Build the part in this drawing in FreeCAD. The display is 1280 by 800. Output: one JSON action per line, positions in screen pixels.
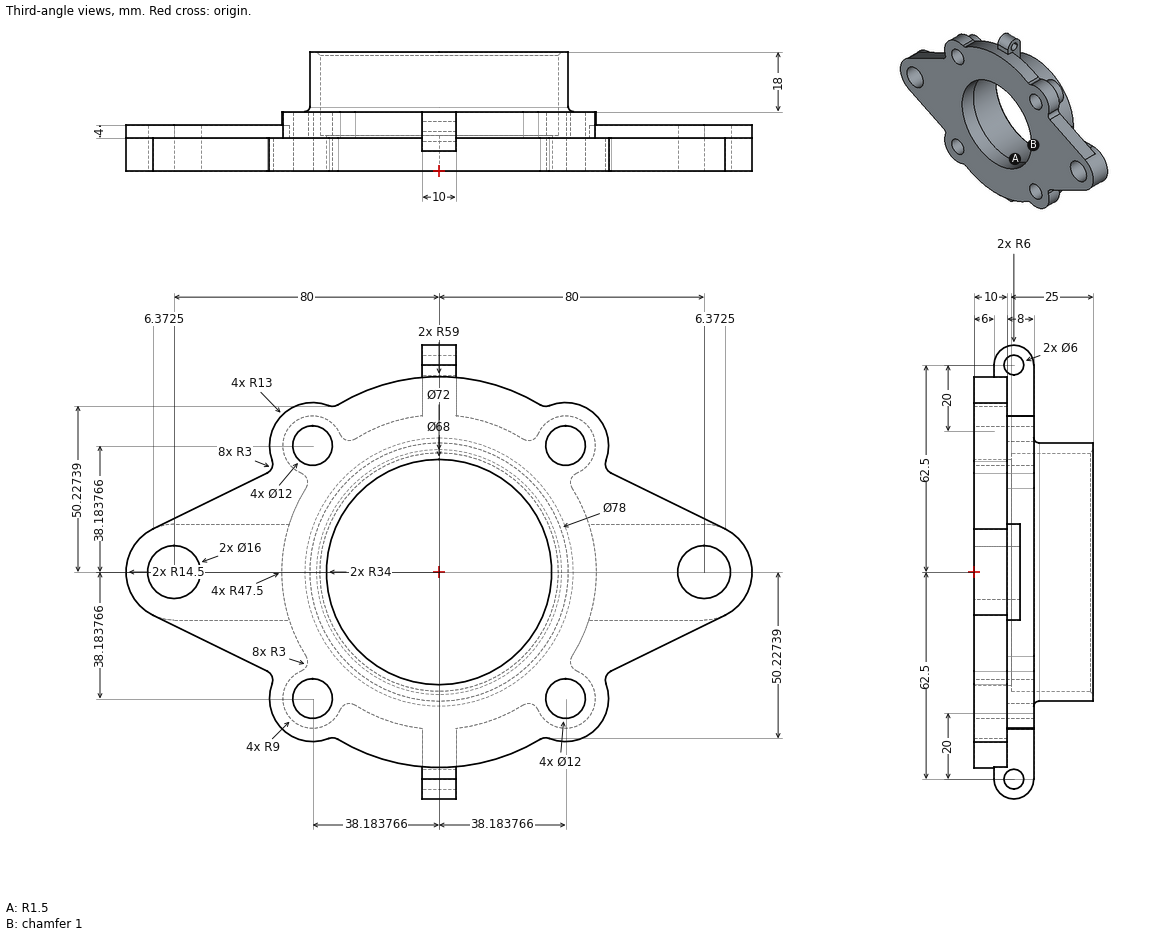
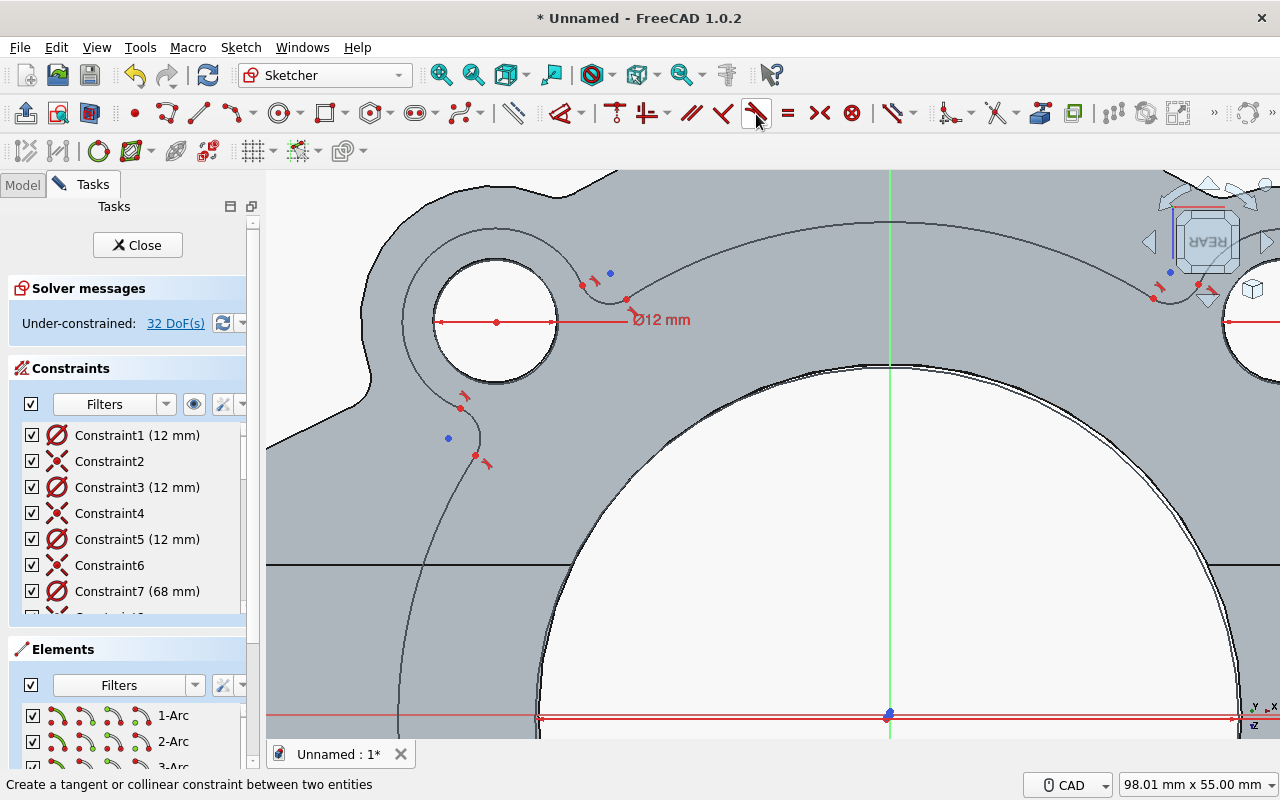
{"action": "left_click", "coordinate": [638, 471]}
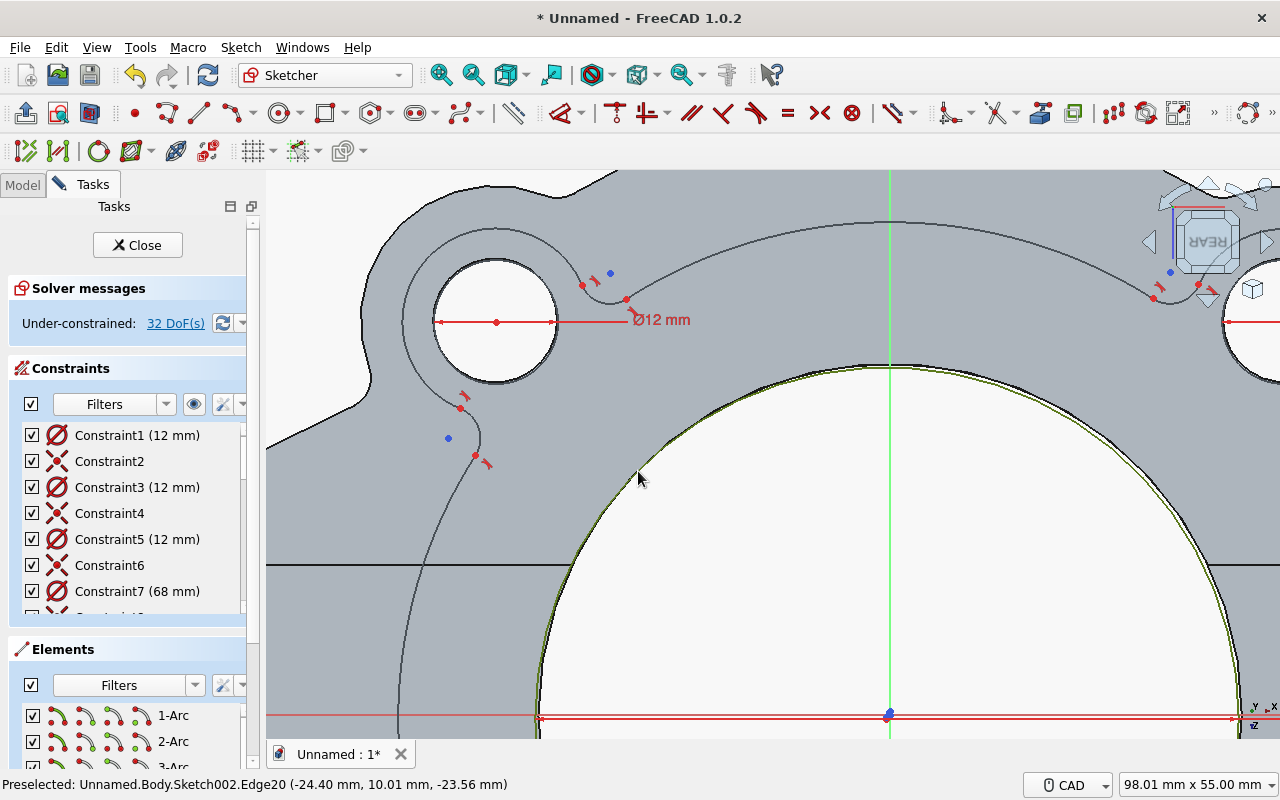
{"action": "scroll", "coordinate": [596, 303], "scroll_direction": "down", "scroll_amount": 5}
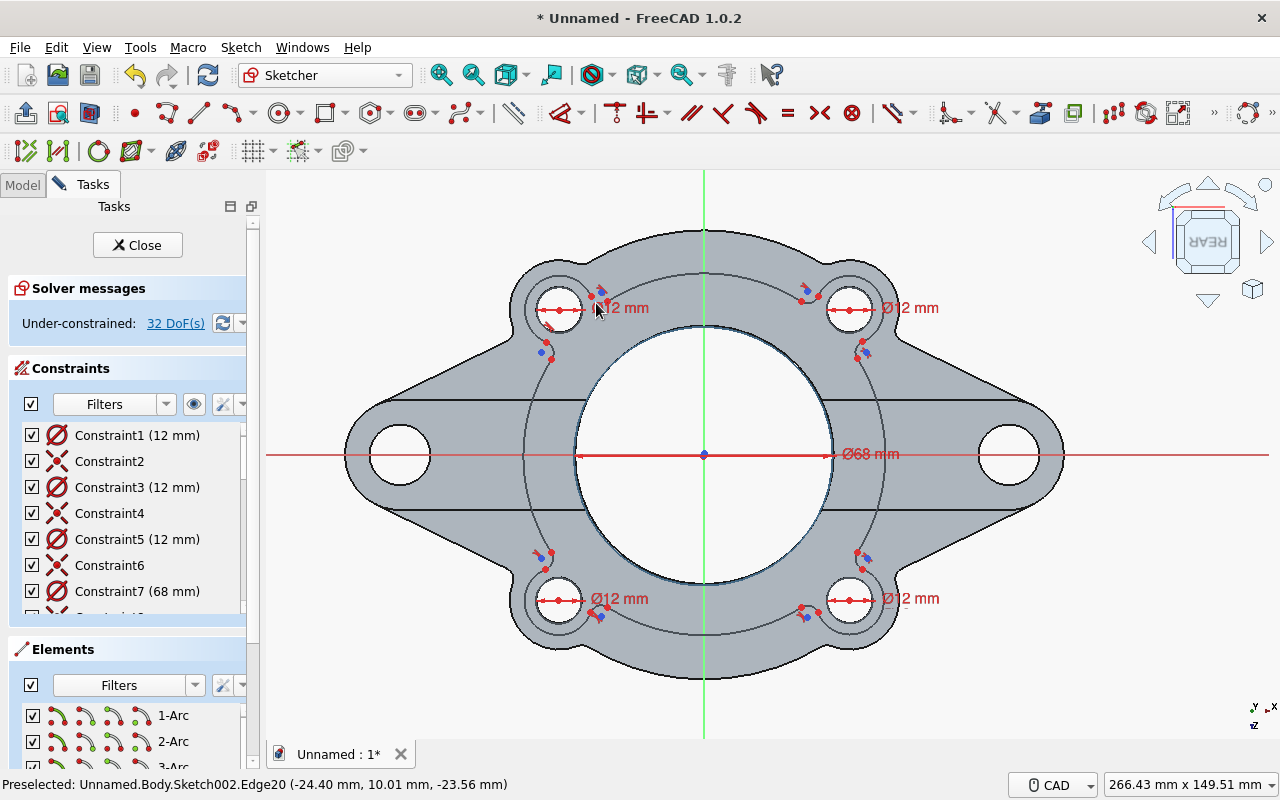
{"action": "left_click", "coordinate": [664, 631]}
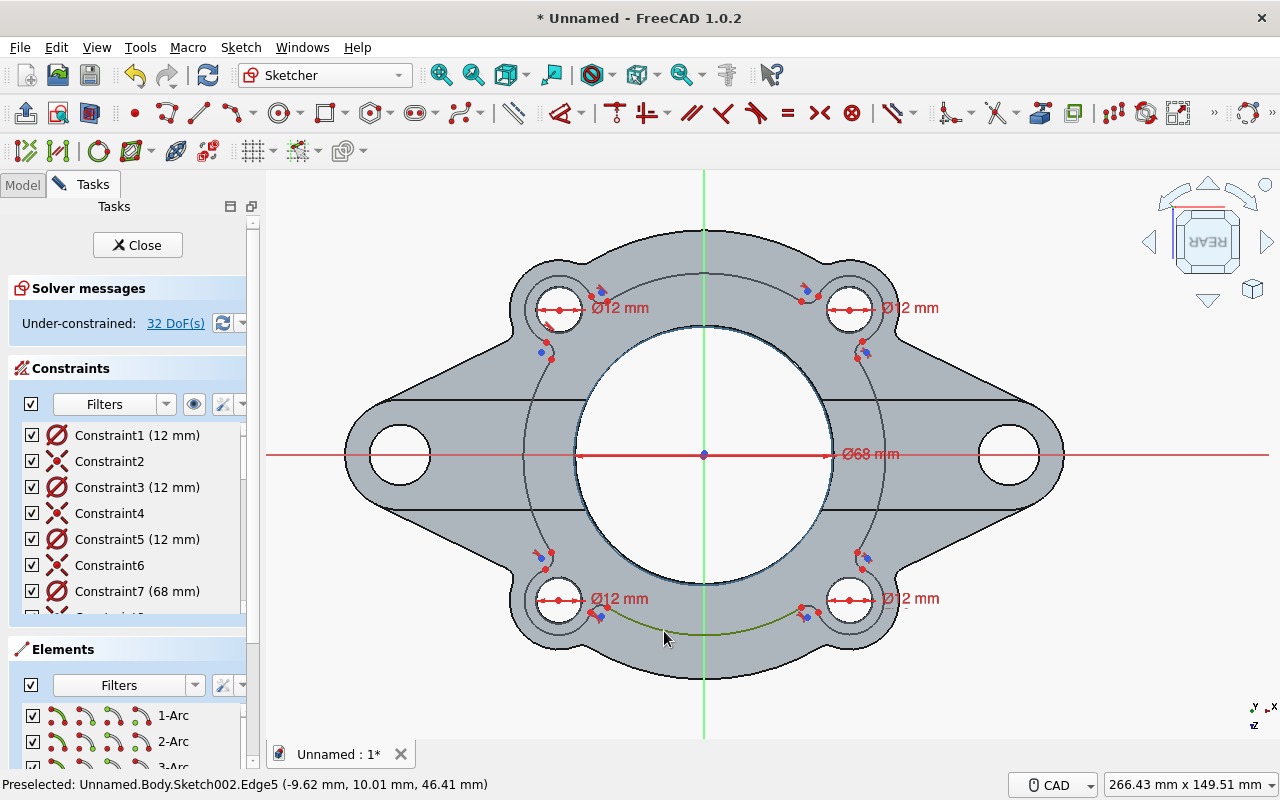
{"action": "left_click", "coordinate": [616, 114]}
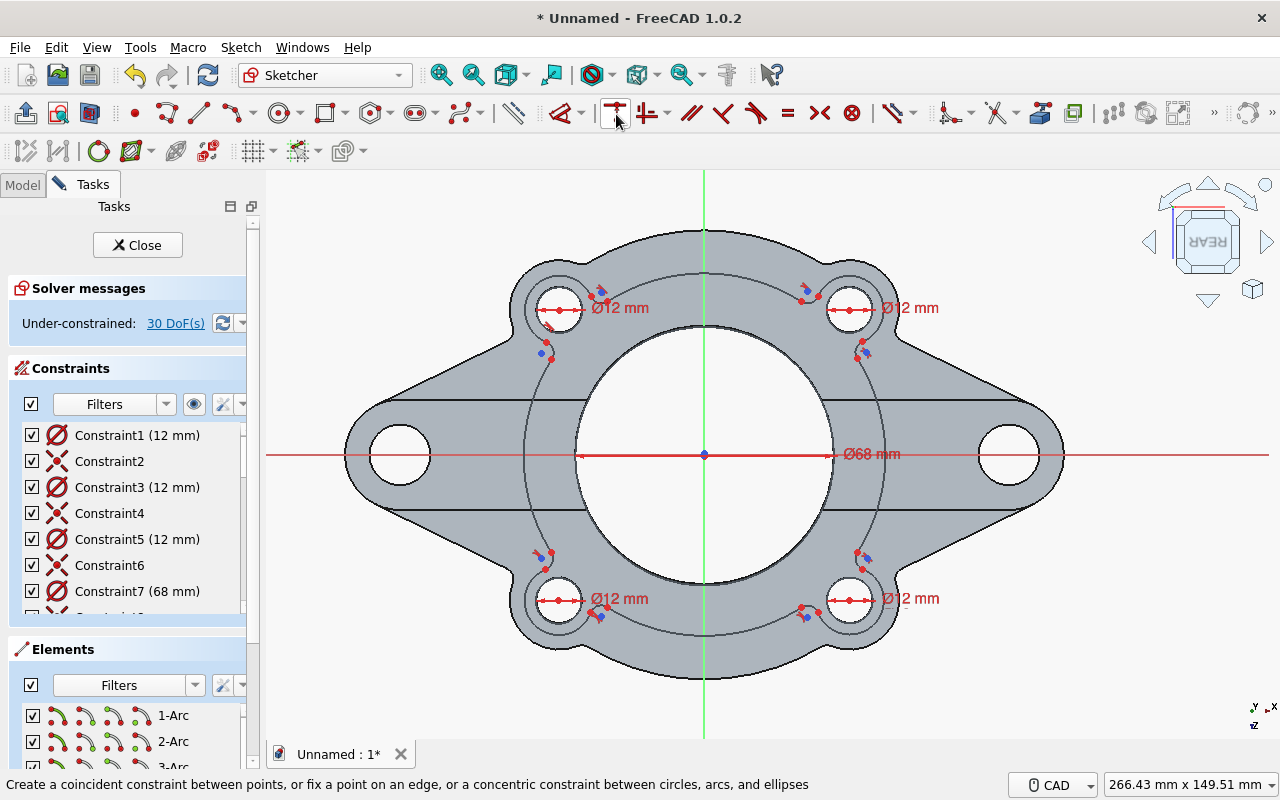
{"action": "left_click", "coordinate": [796, 364]}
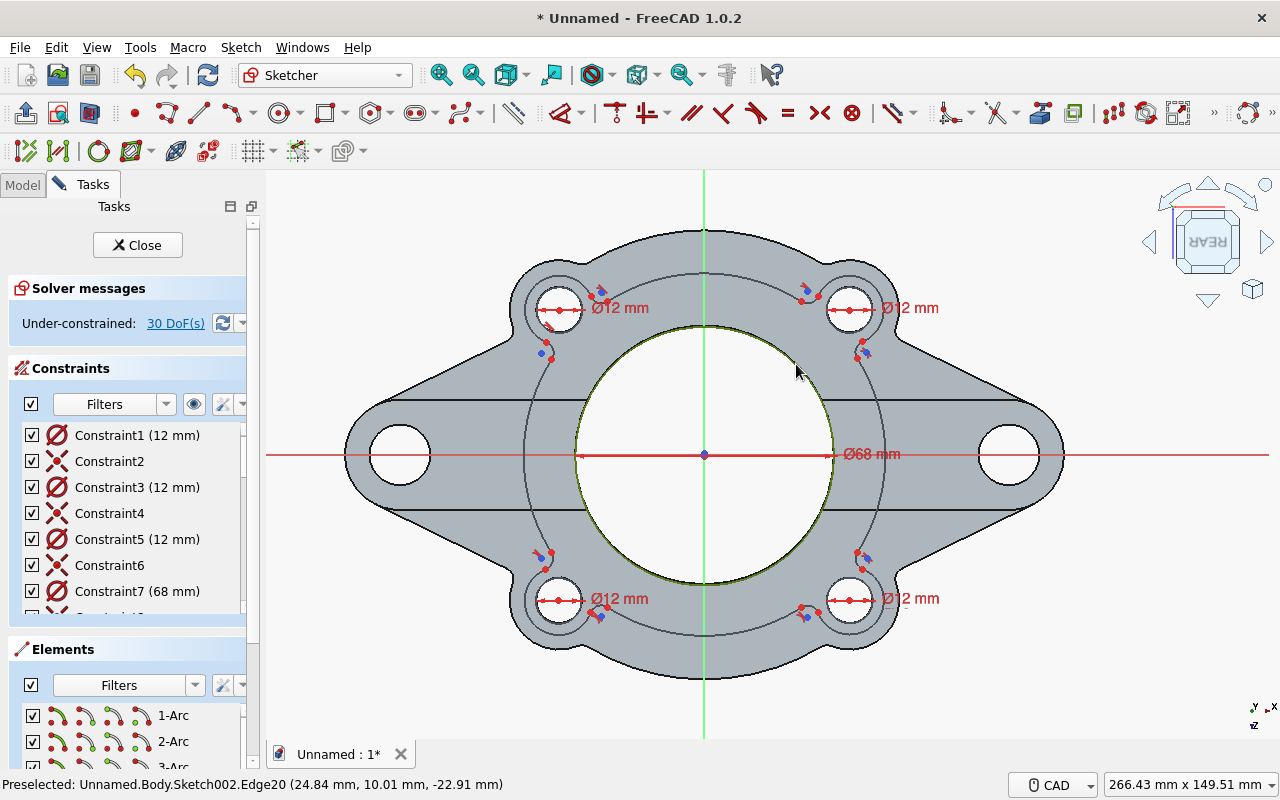
{"action": "left_click", "coordinate": [881, 496]}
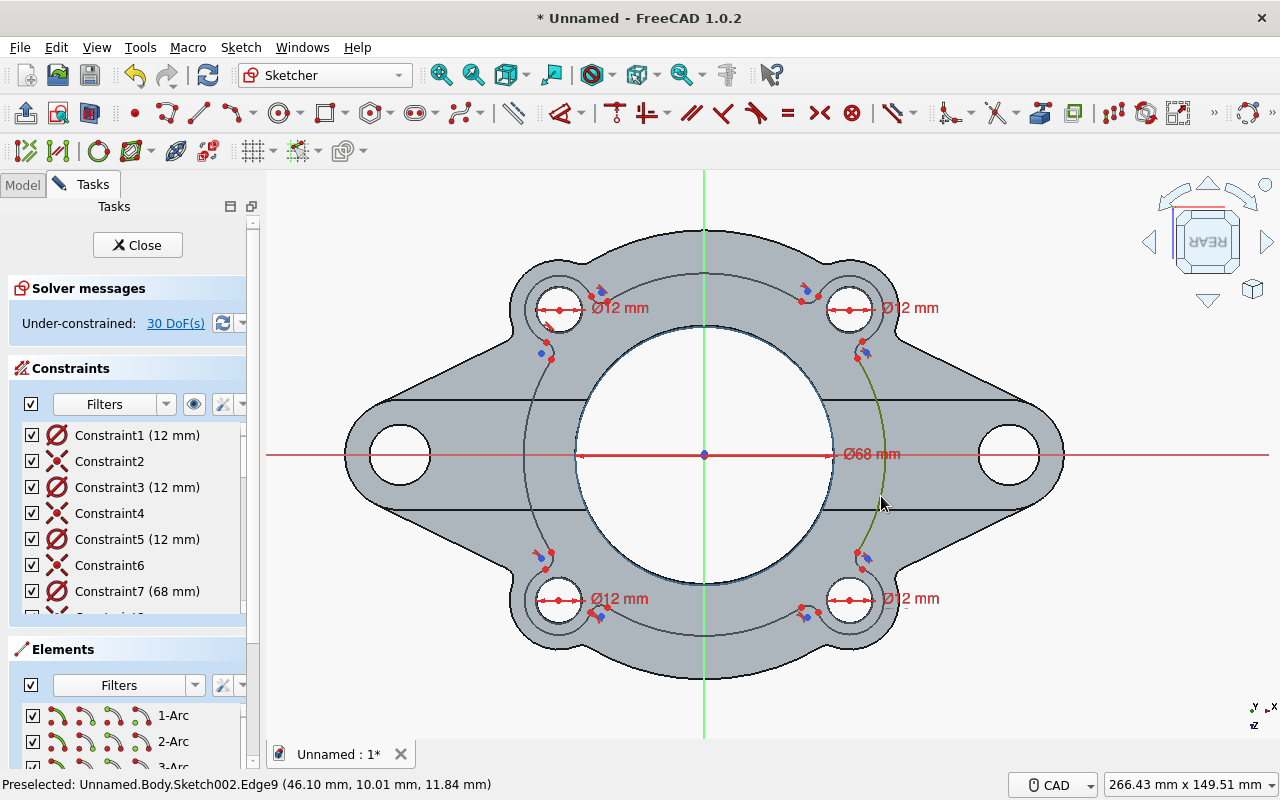
{"action": "left_click", "coordinate": [616, 114]}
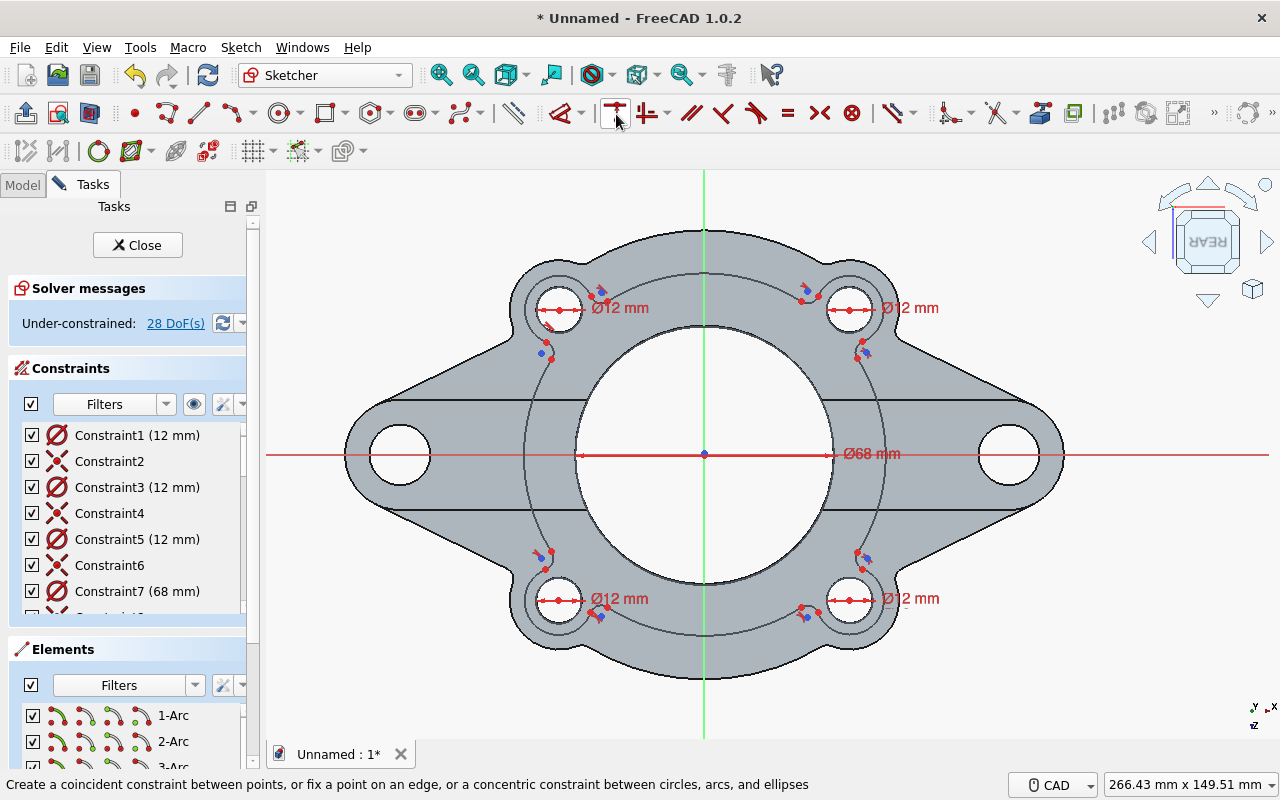
{"action": "left_click", "coordinate": [796, 364]}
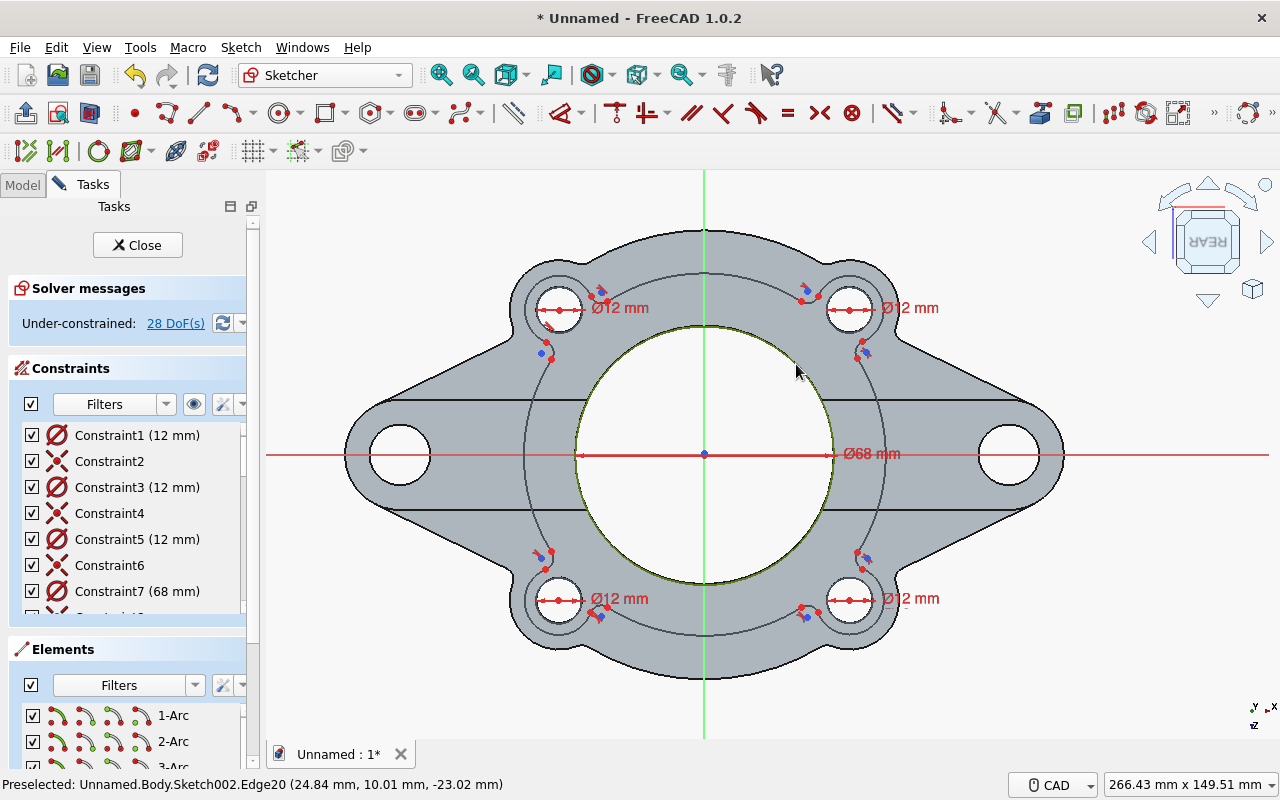
{"action": "left_click", "coordinate": [745, 278]}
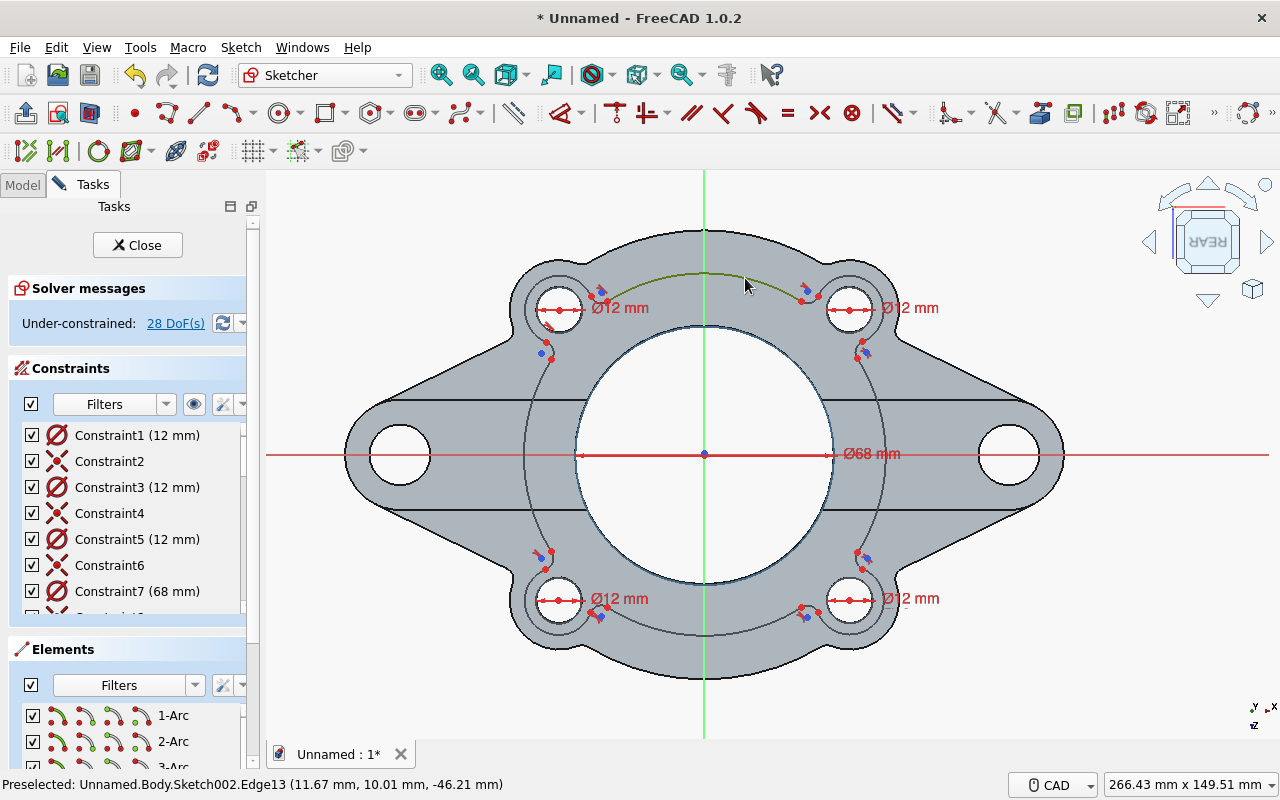
{"action": "left_click", "coordinate": [616, 114]}